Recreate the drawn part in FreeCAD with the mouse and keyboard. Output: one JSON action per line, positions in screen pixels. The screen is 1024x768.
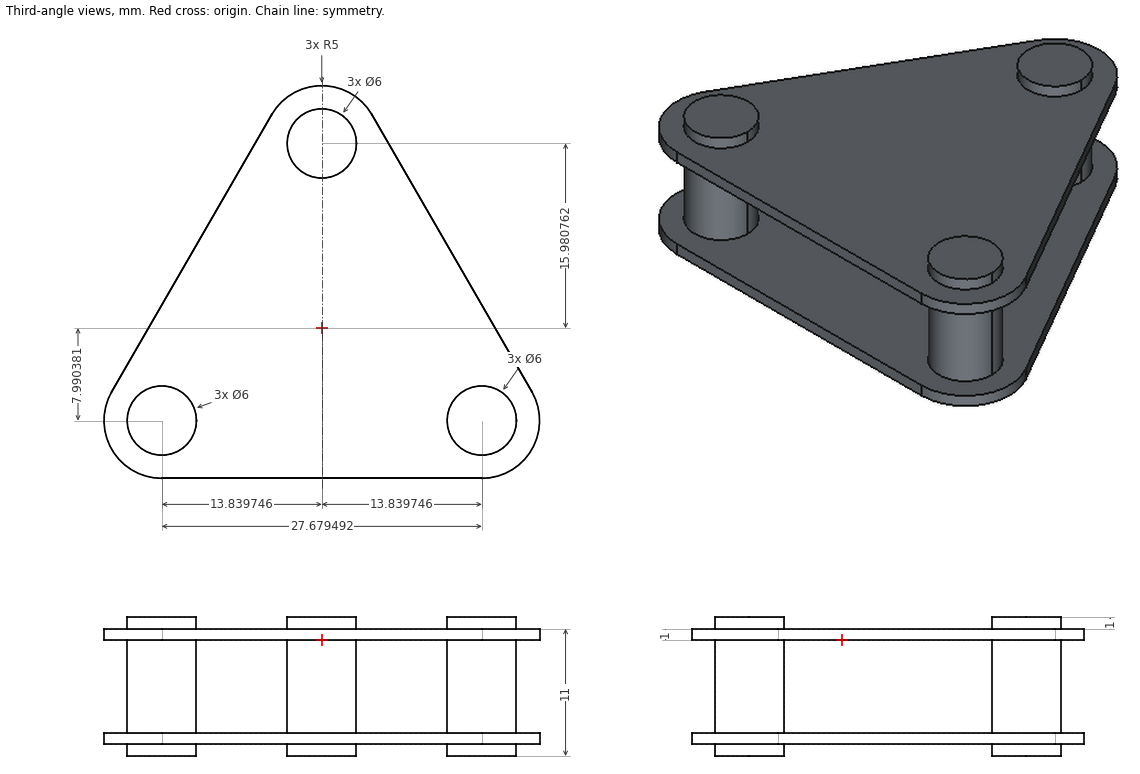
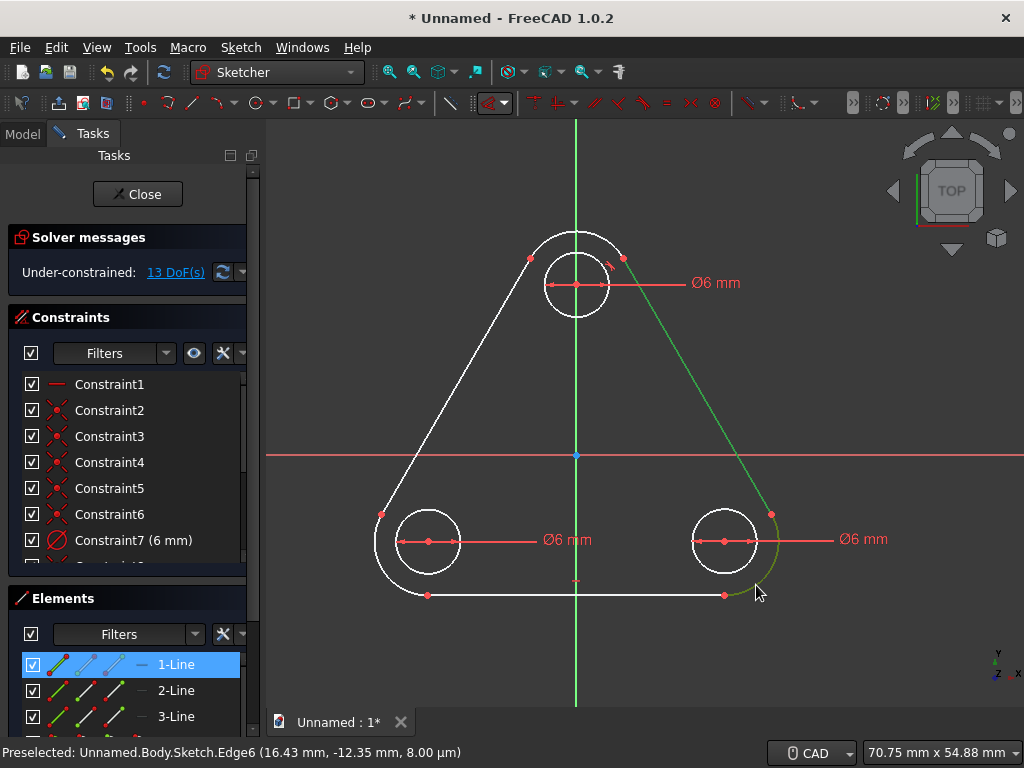
{"action": "left_click", "coordinate": [644, 104]}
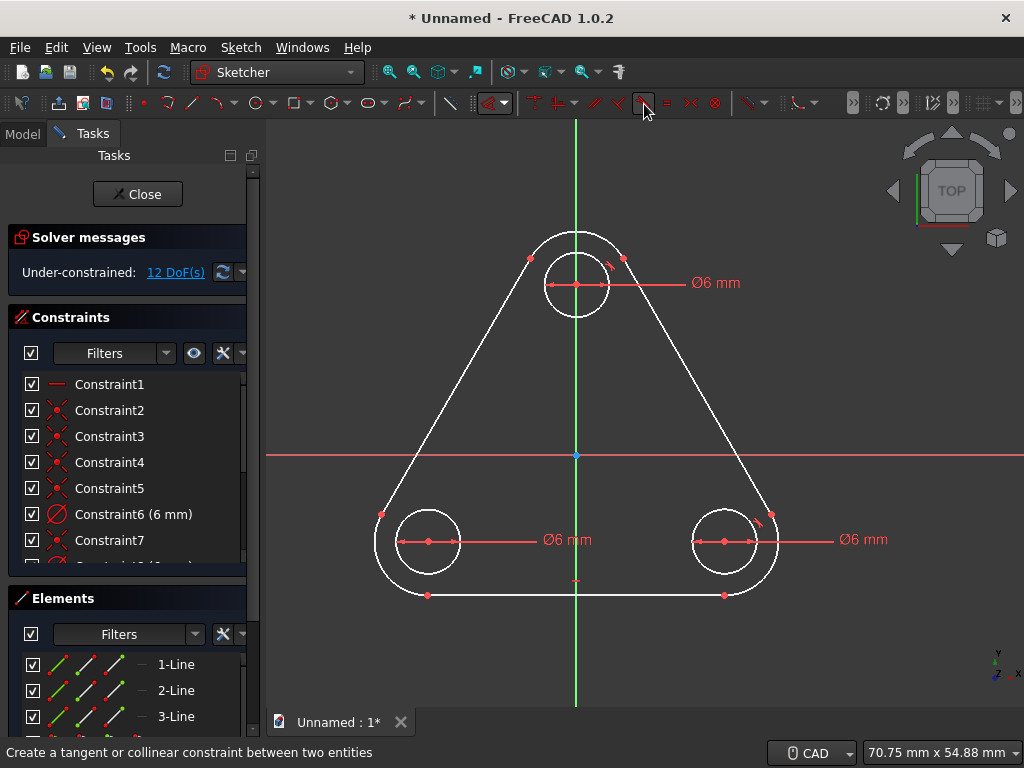
{"action": "left_click", "coordinate": [486, 335]}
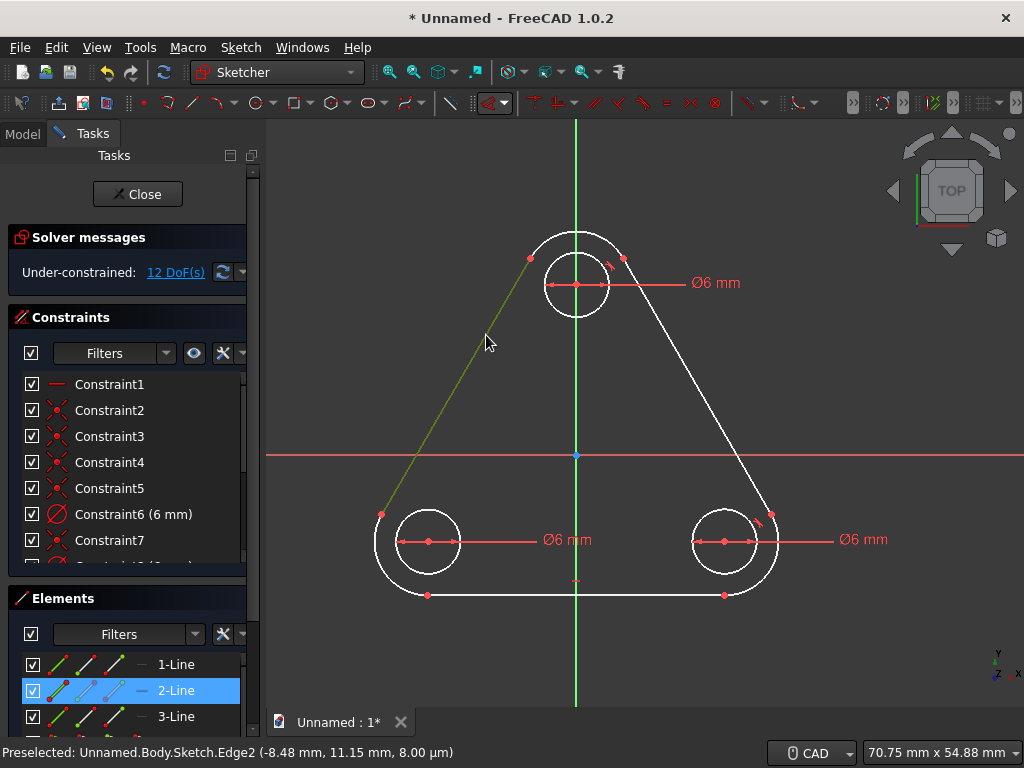
{"action": "left_click", "coordinate": [598, 236]}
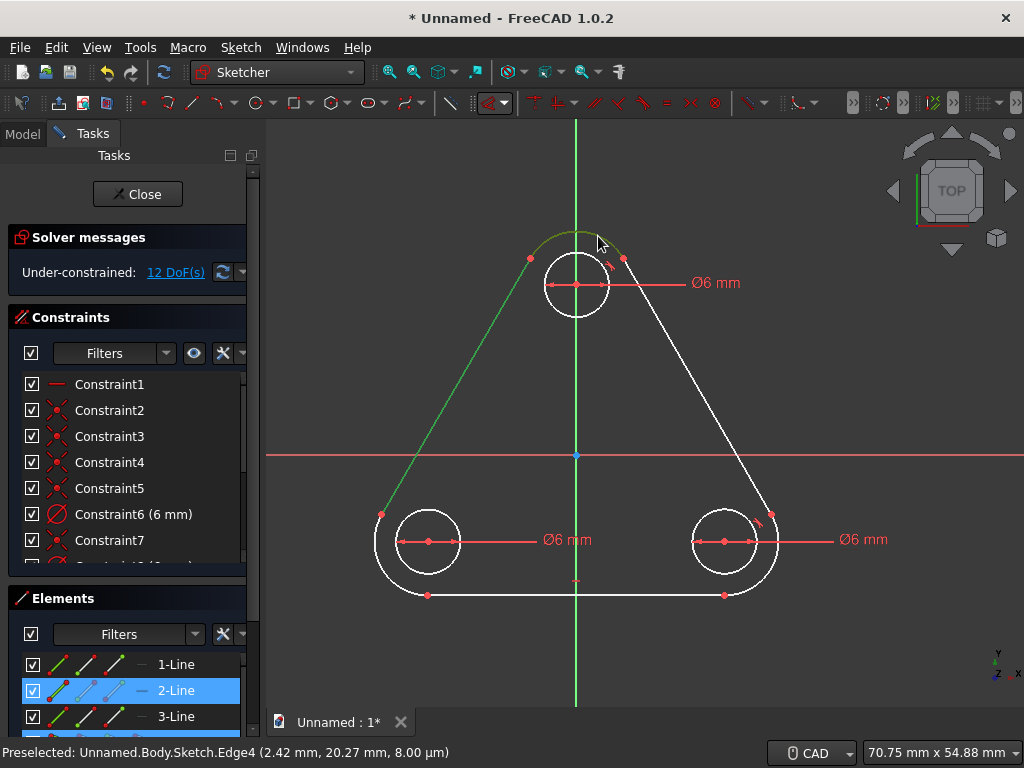
{"action": "left_click", "coordinate": [644, 104]}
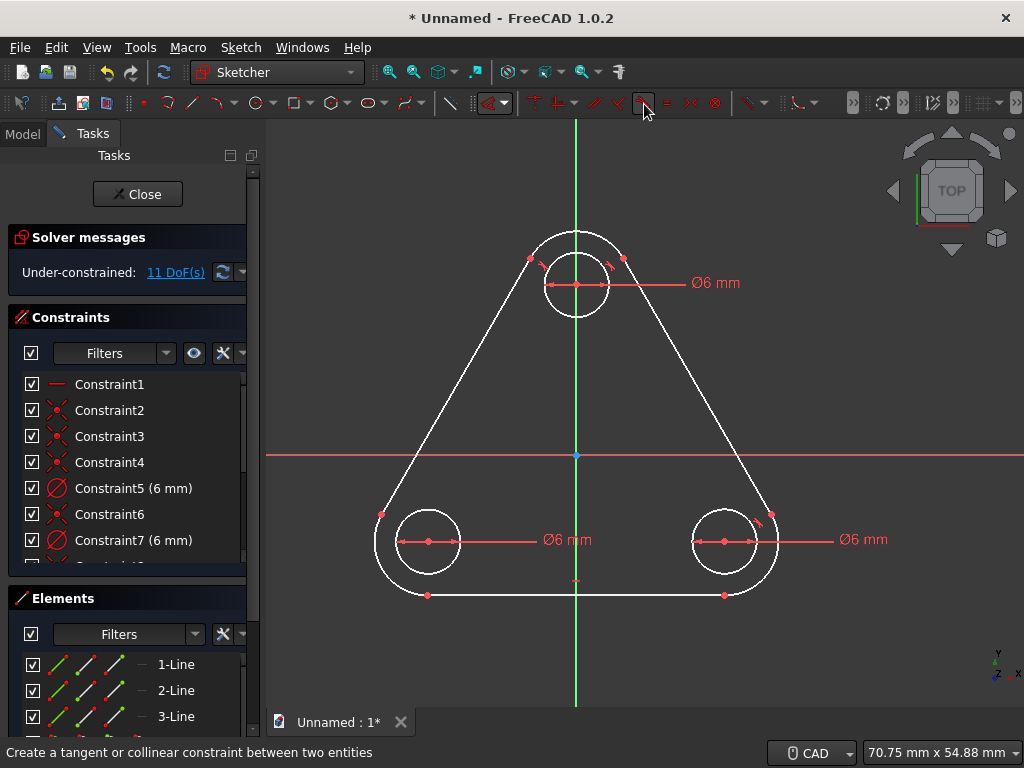
{"action": "left_click", "coordinate": [486, 335]}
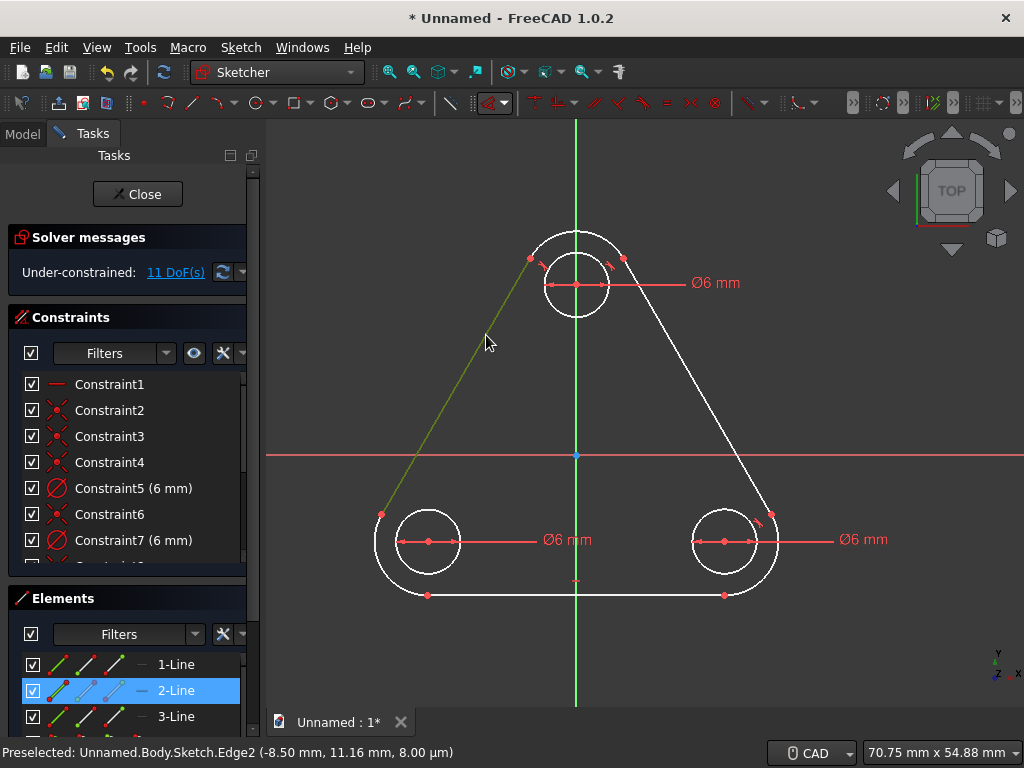
{"action": "left_click", "coordinate": [375, 547]}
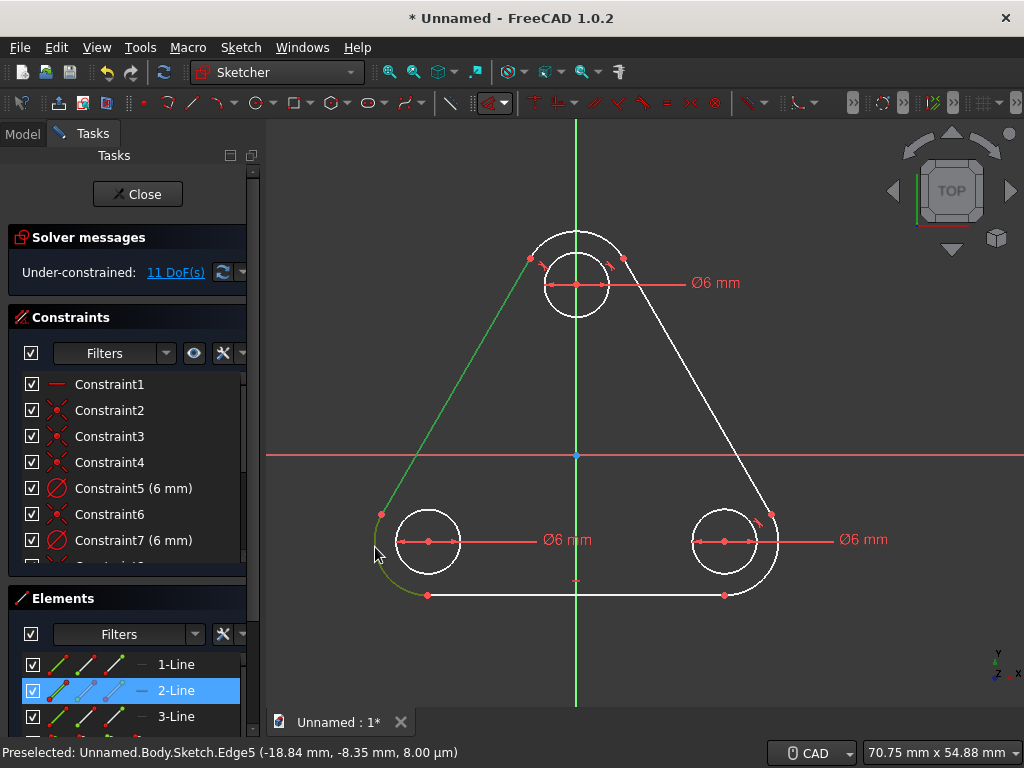
{"action": "left_click", "coordinate": [644, 104]}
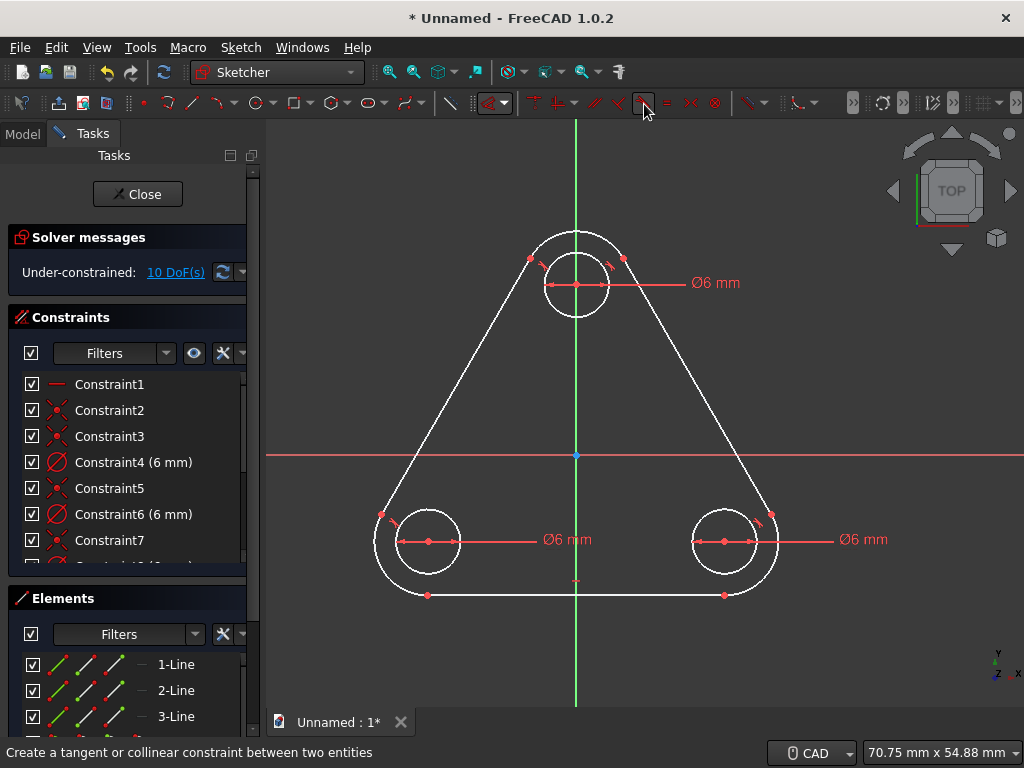
{"action": "left_click", "coordinate": [517, 595]}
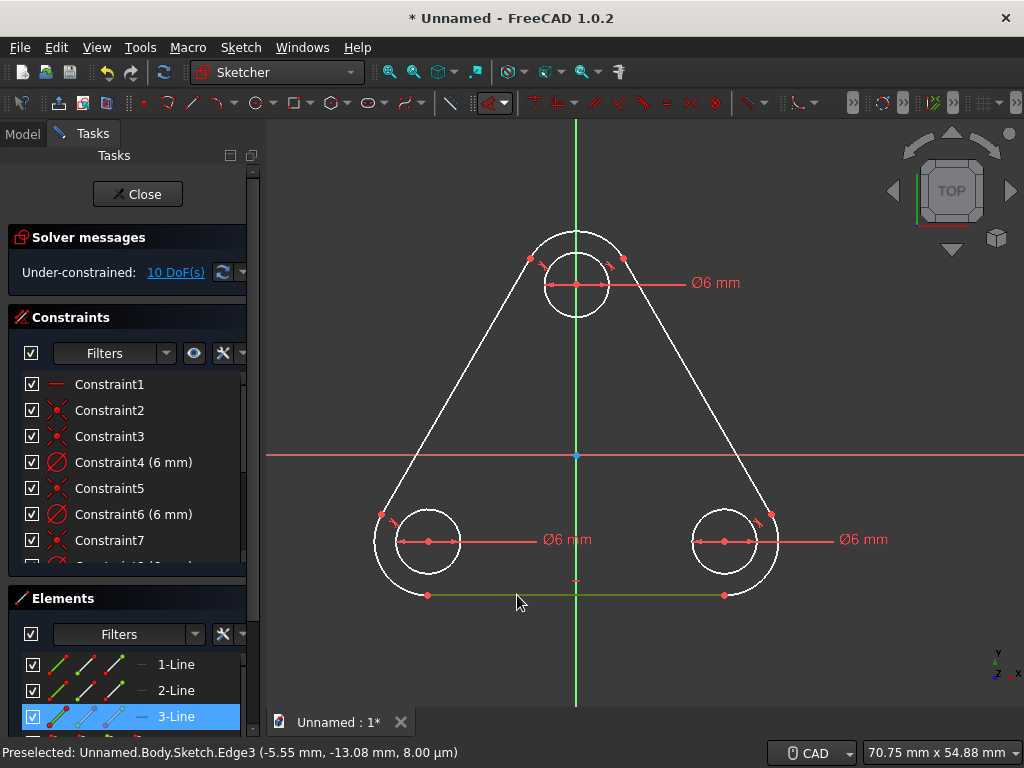
{"action": "left_click", "coordinate": [375, 547]}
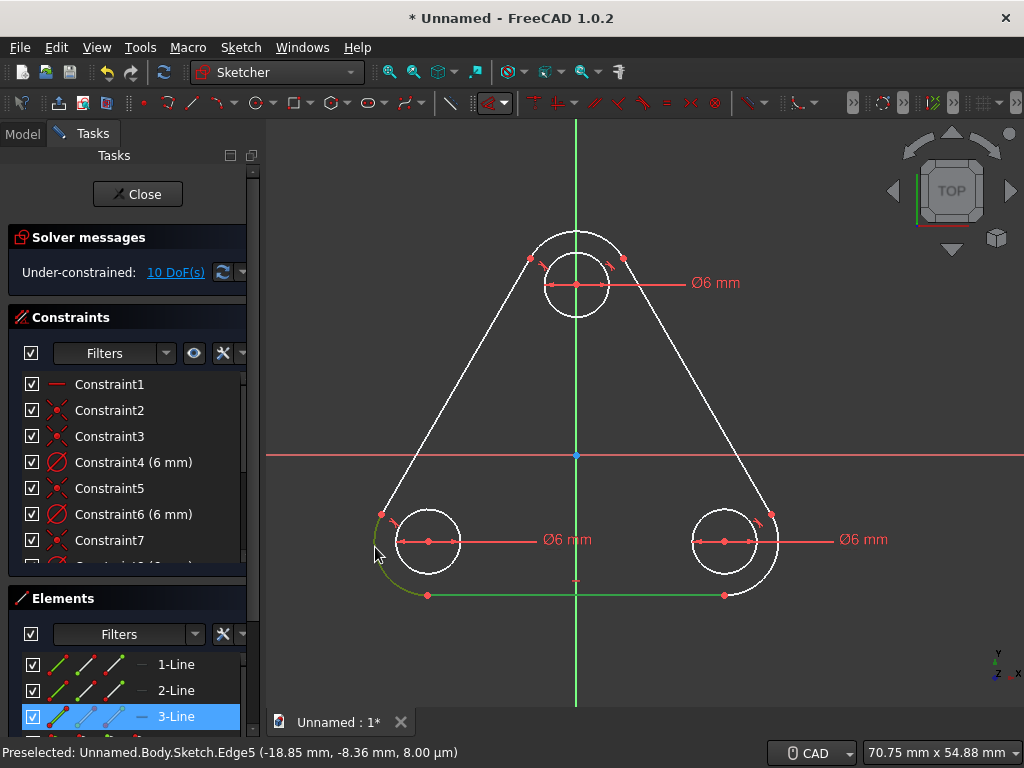
{"action": "left_click", "coordinate": [644, 104]}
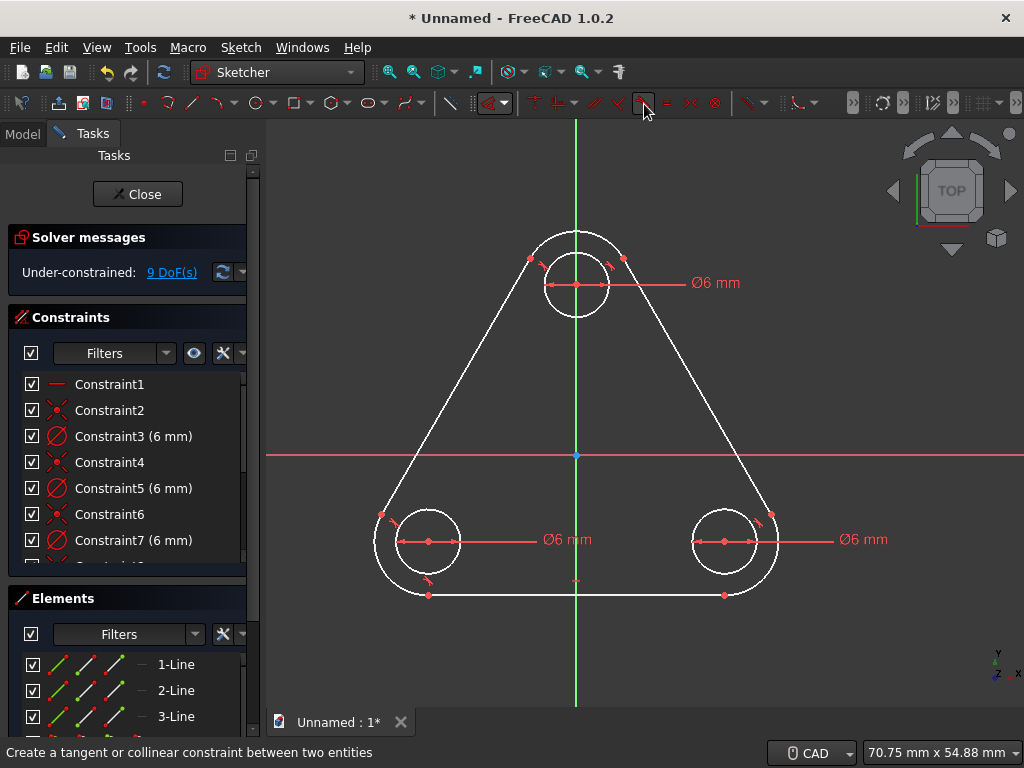
{"action": "left_click", "coordinate": [517, 595]}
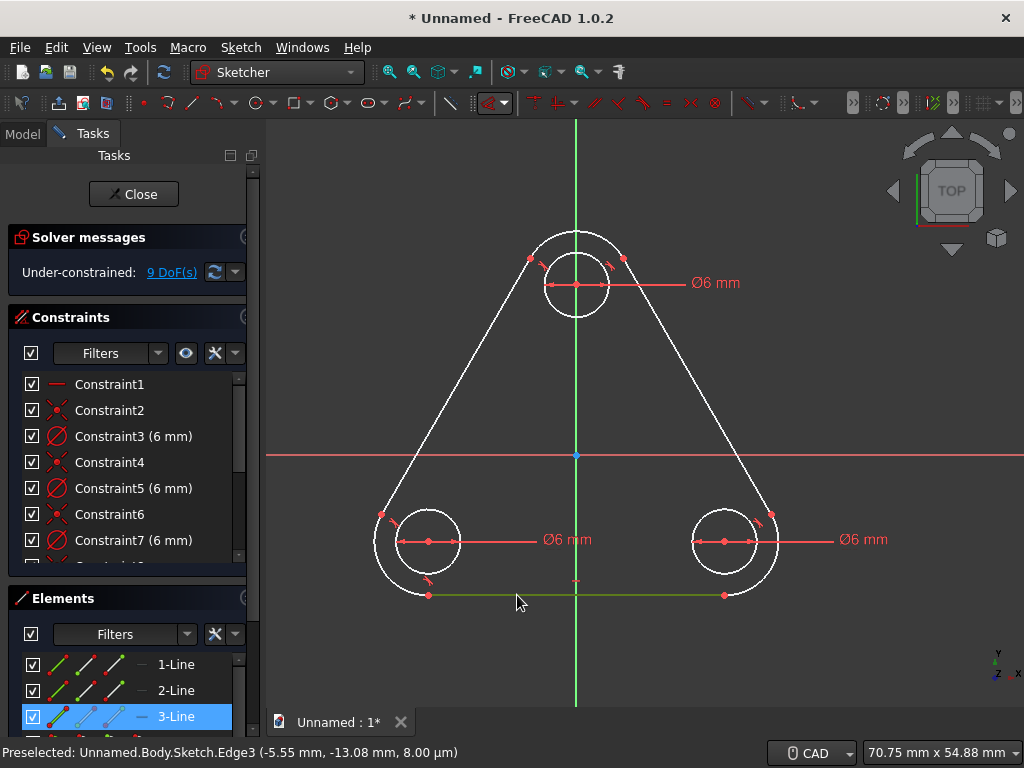
{"action": "left_click", "coordinate": [756, 585]}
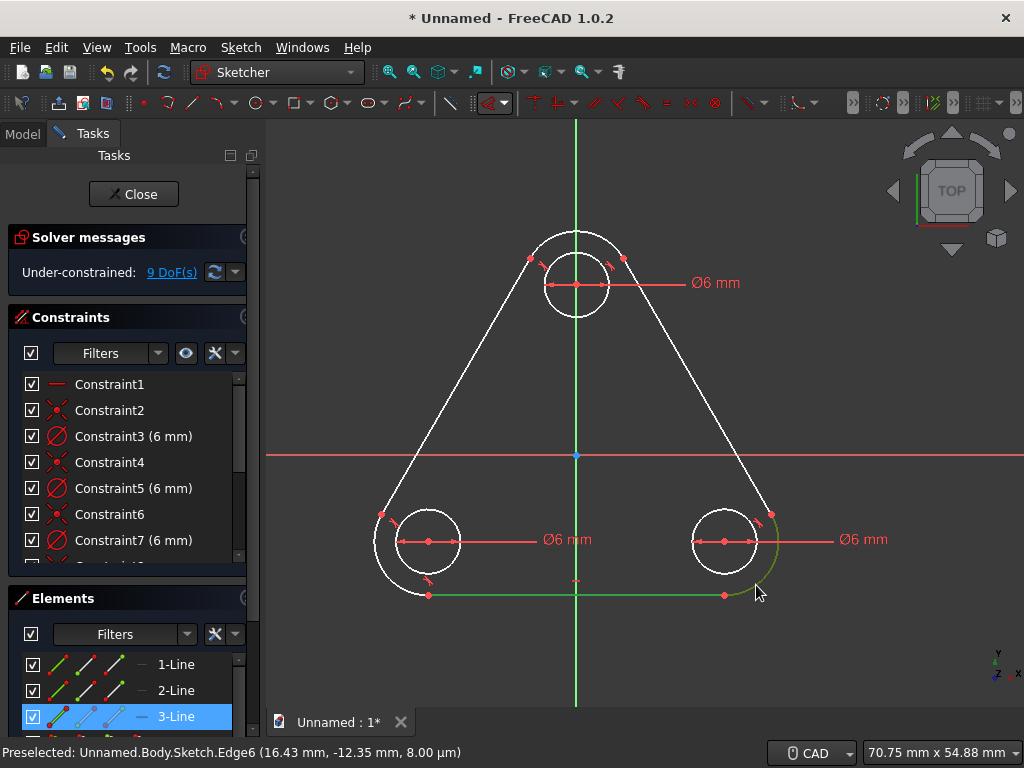
{"action": "left_click", "coordinate": [644, 104]}